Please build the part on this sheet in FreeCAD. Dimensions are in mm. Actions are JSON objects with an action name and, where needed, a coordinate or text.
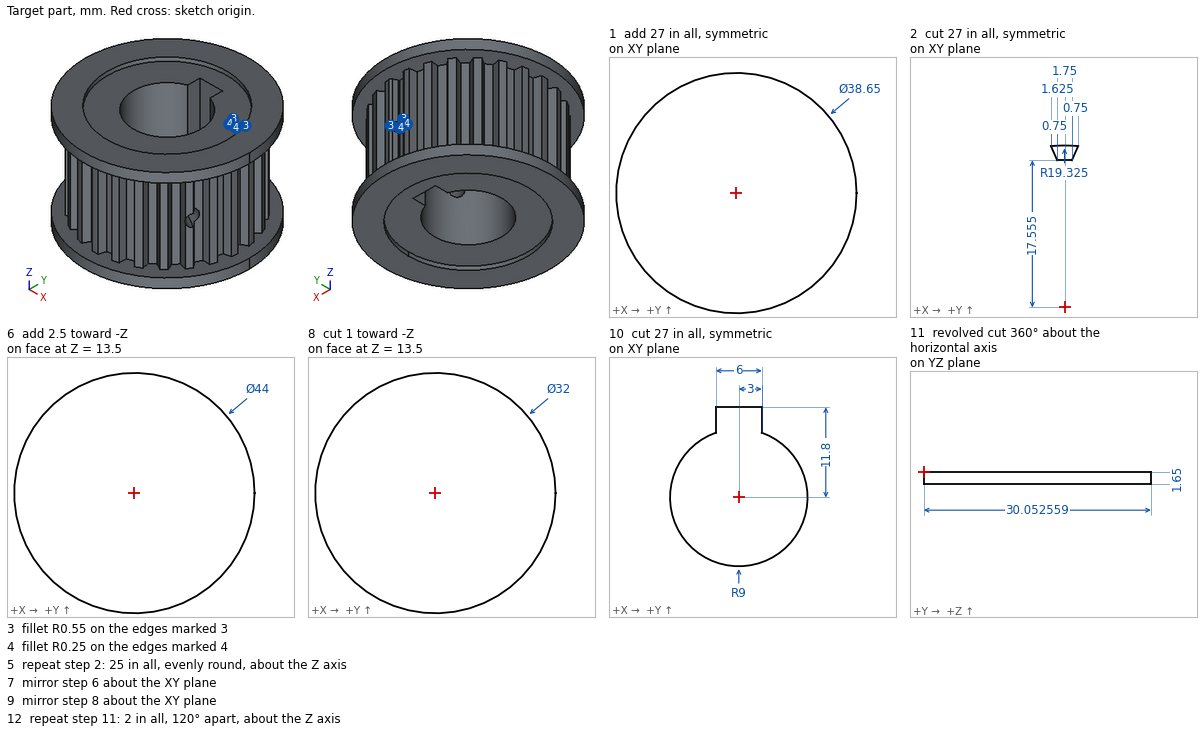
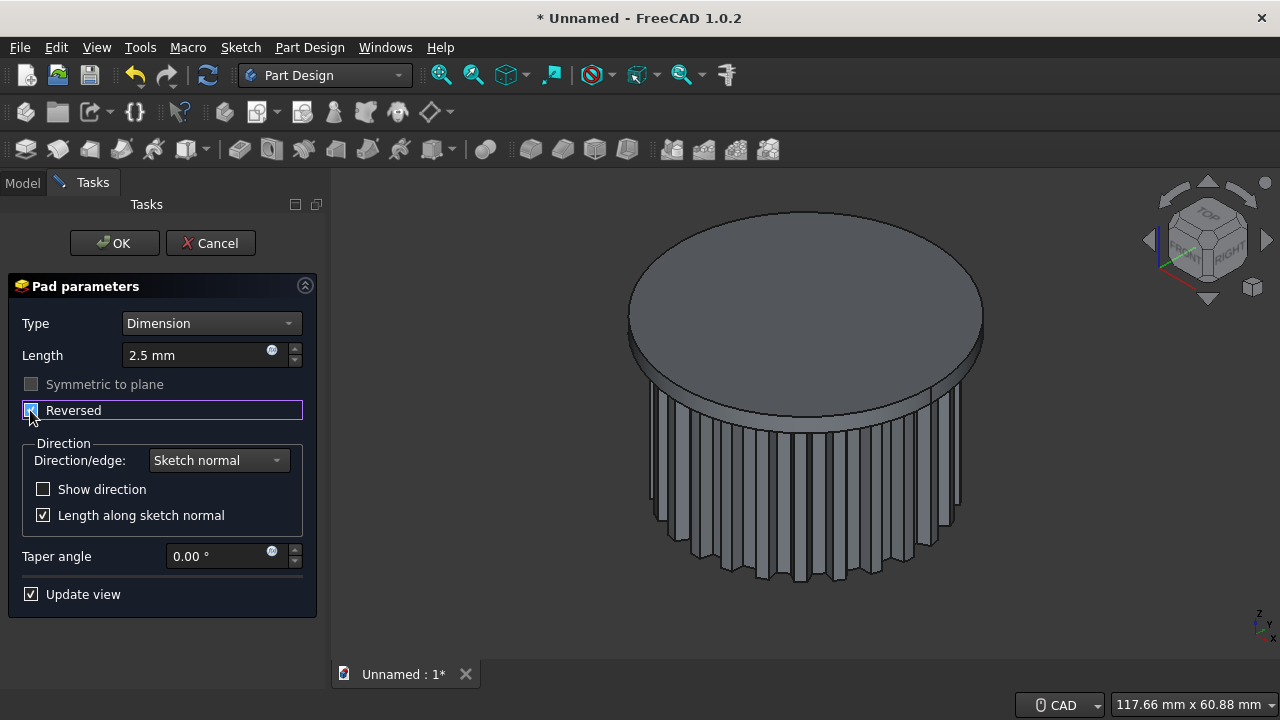
{"action": "left_click", "coordinate": [115, 243]}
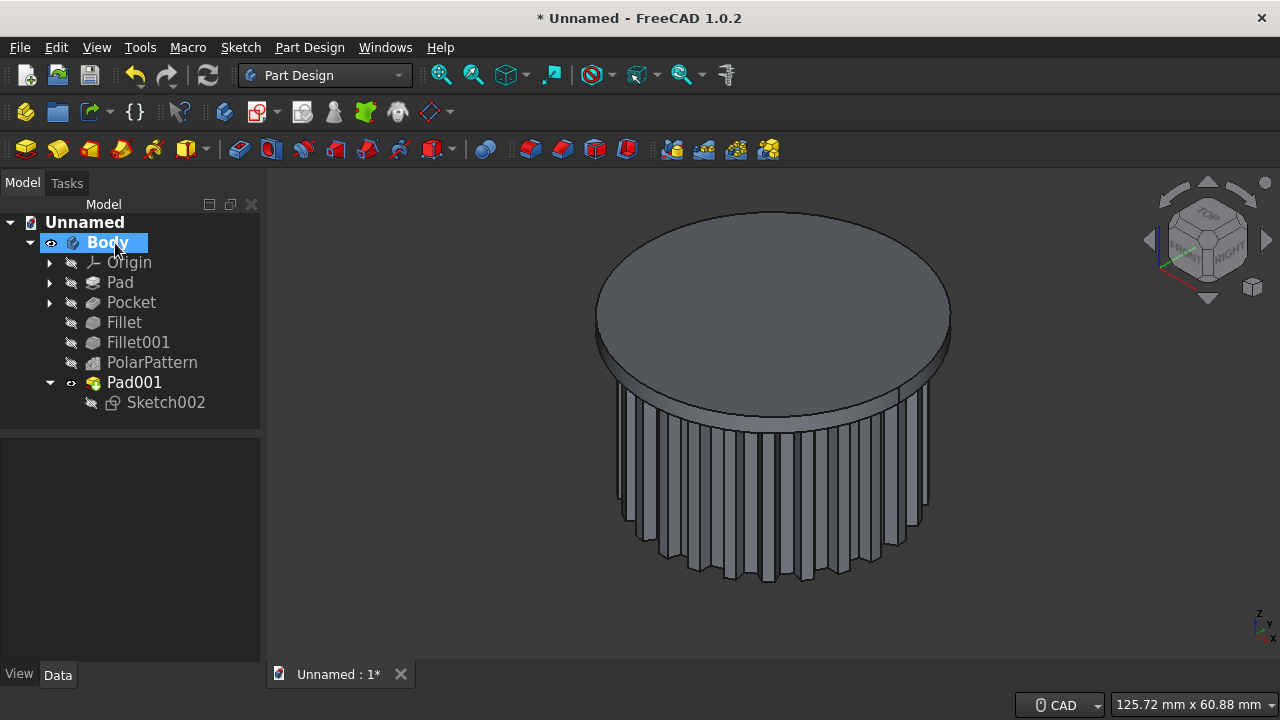
{"action": "left_click", "coordinate": [116, 383]}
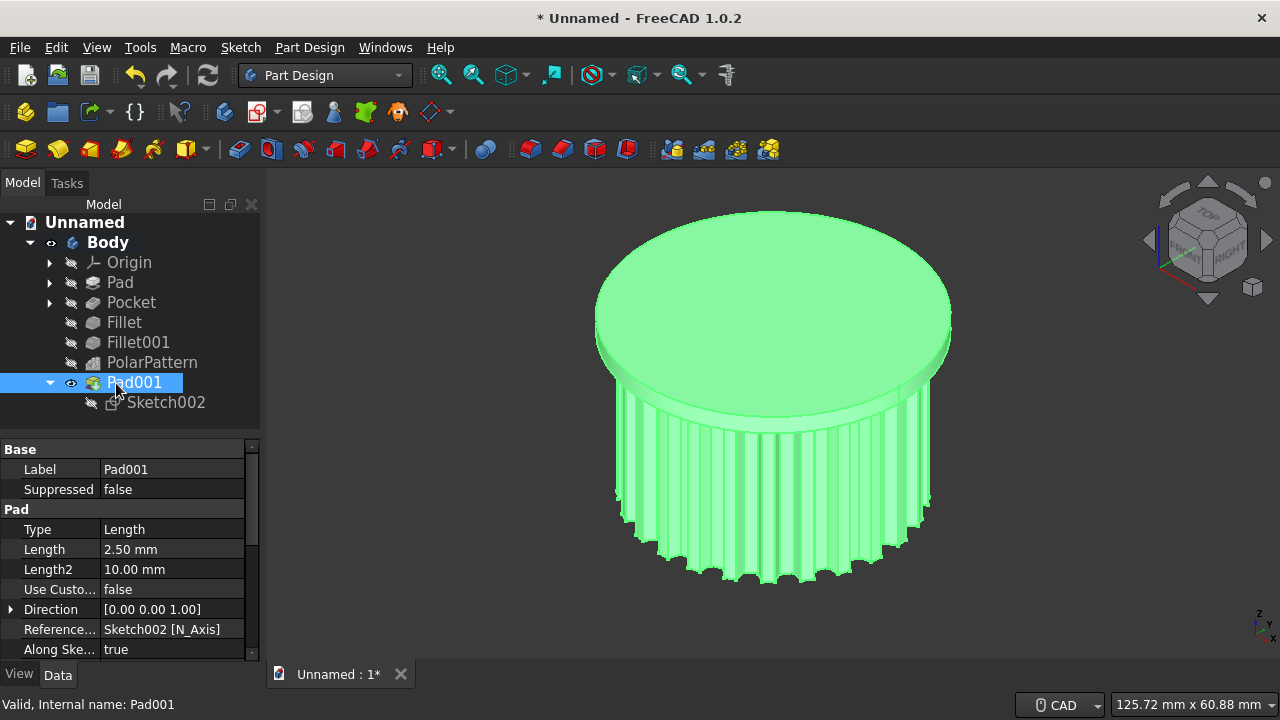
{"action": "left_click", "coordinate": [672, 150]}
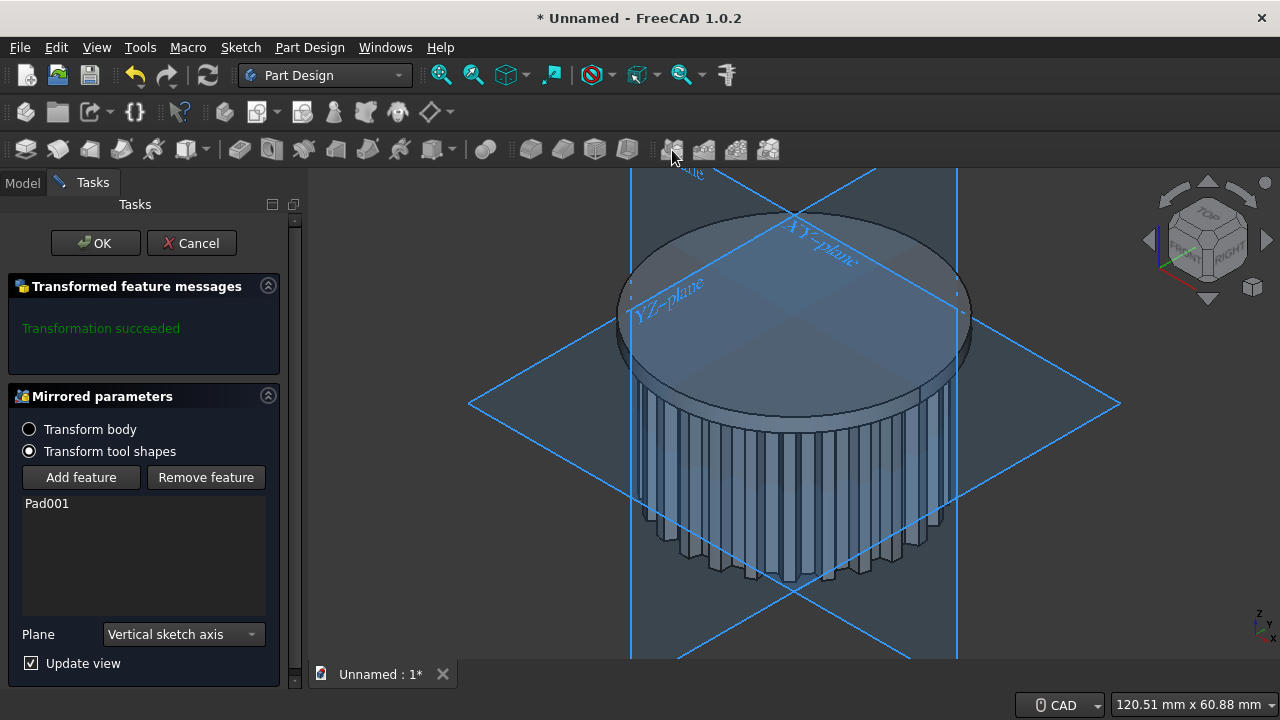
{"action": "left_click", "coordinate": [184, 634]}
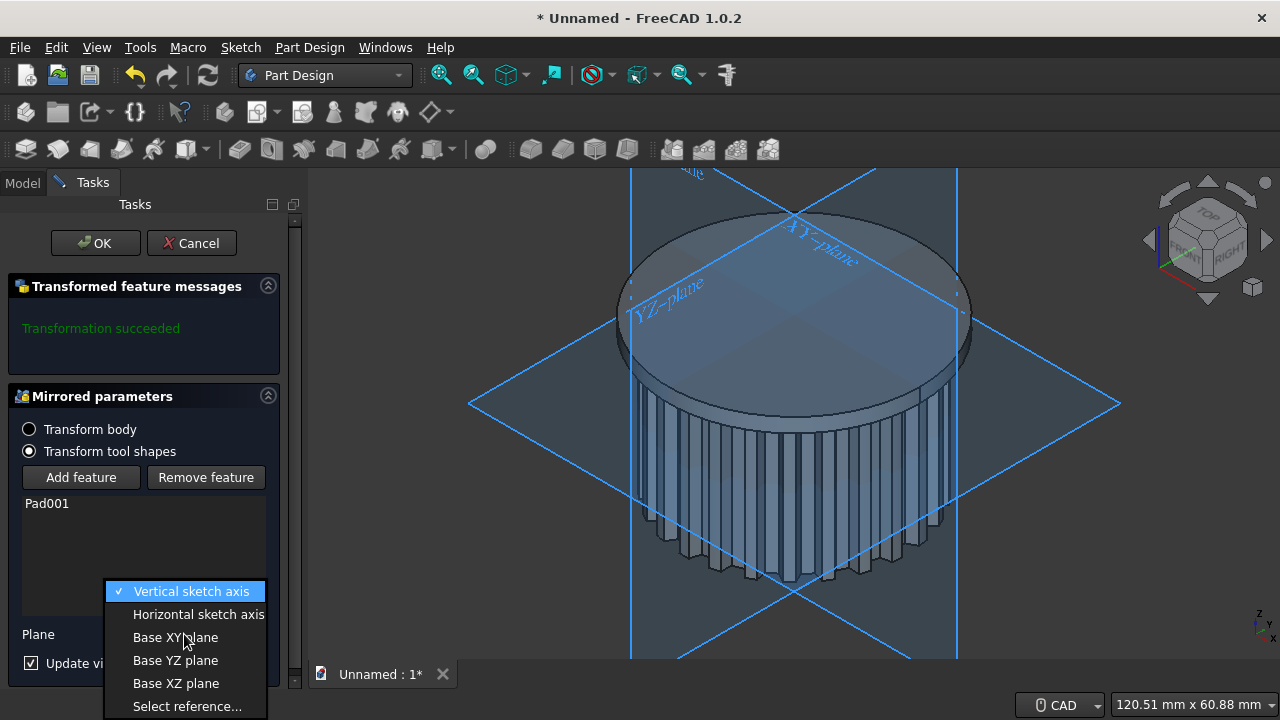
{"action": "left_click", "coordinate": [184, 638]}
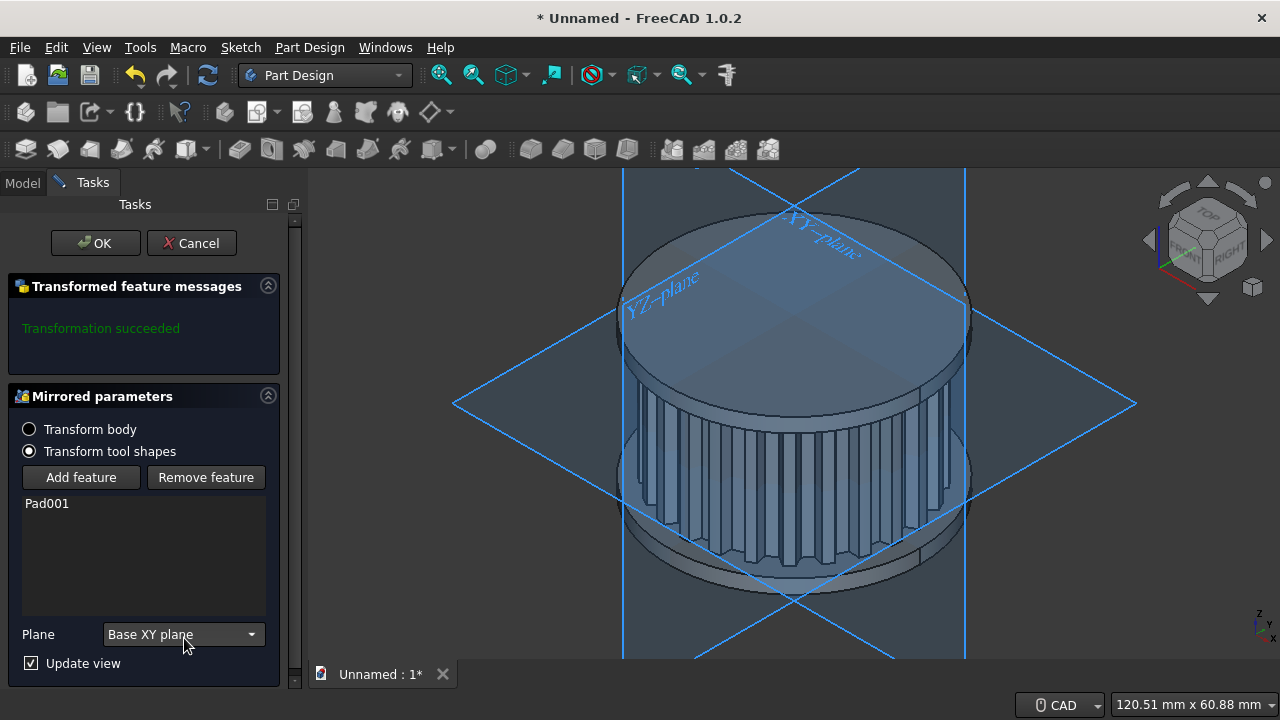
{"action": "left_click", "coordinate": [96, 243]}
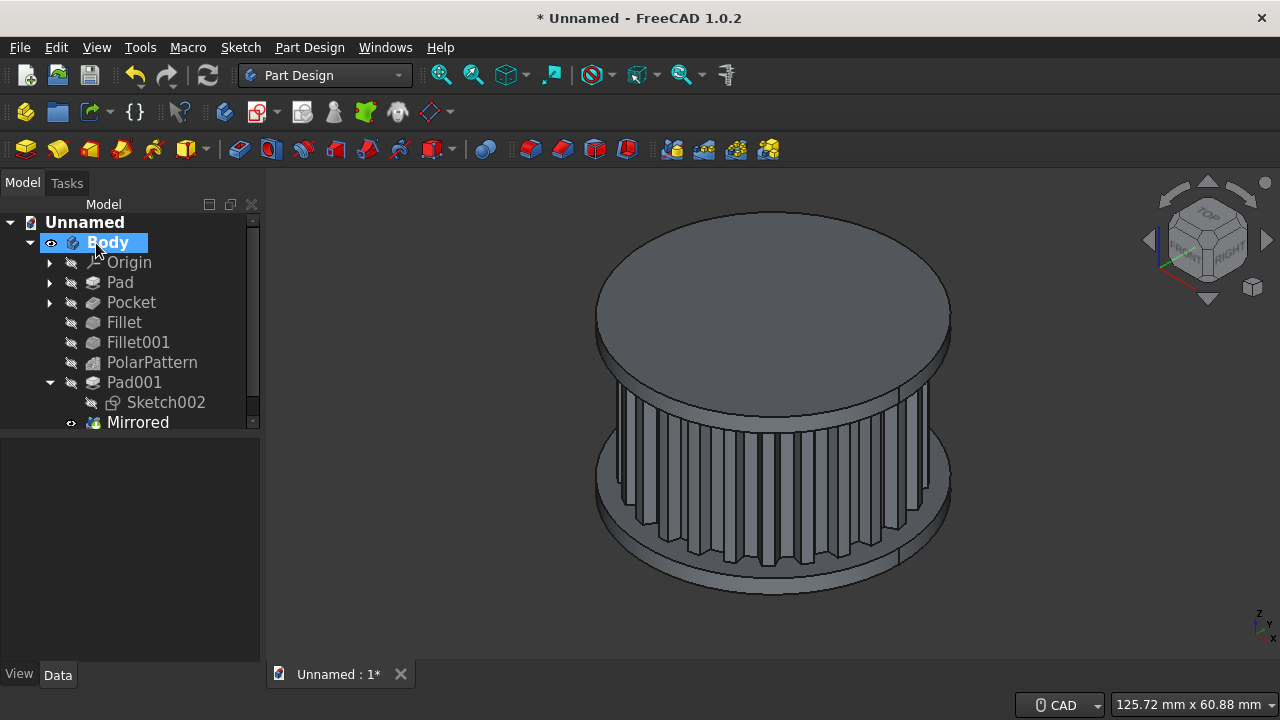
{"action": "left_click", "coordinate": [773, 314]}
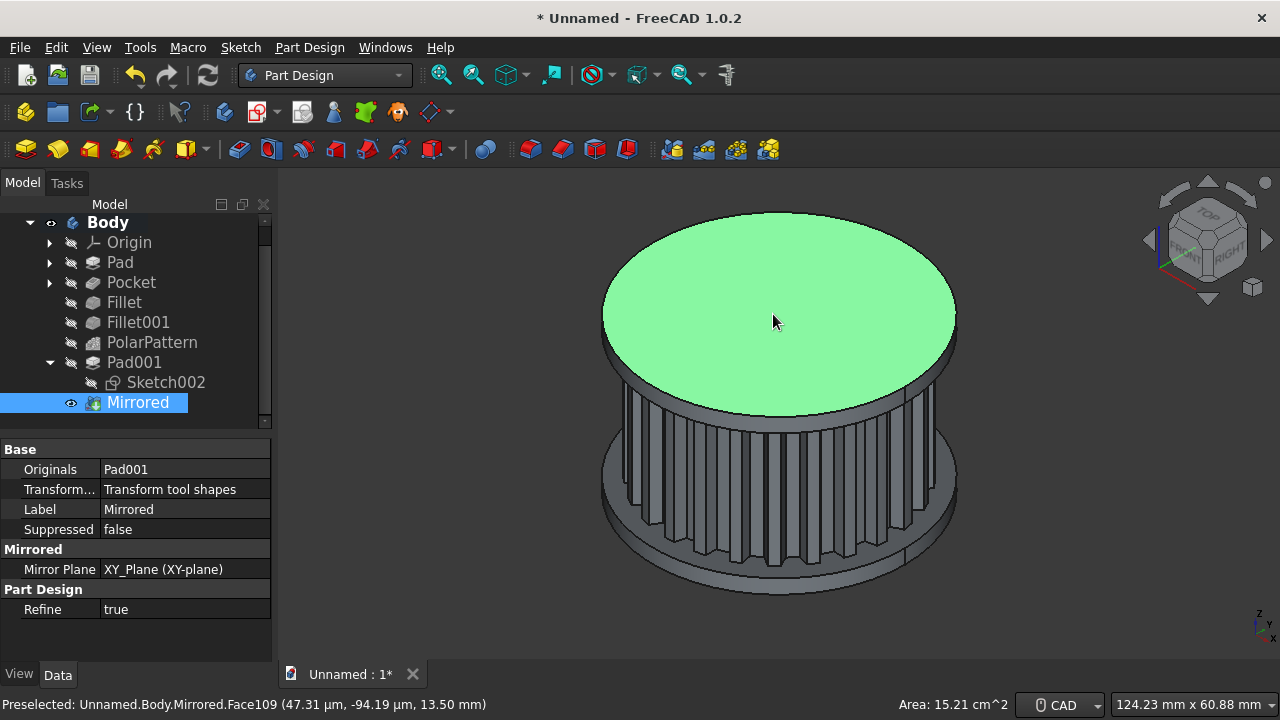
{"action": "left_click", "coordinate": [258, 112]}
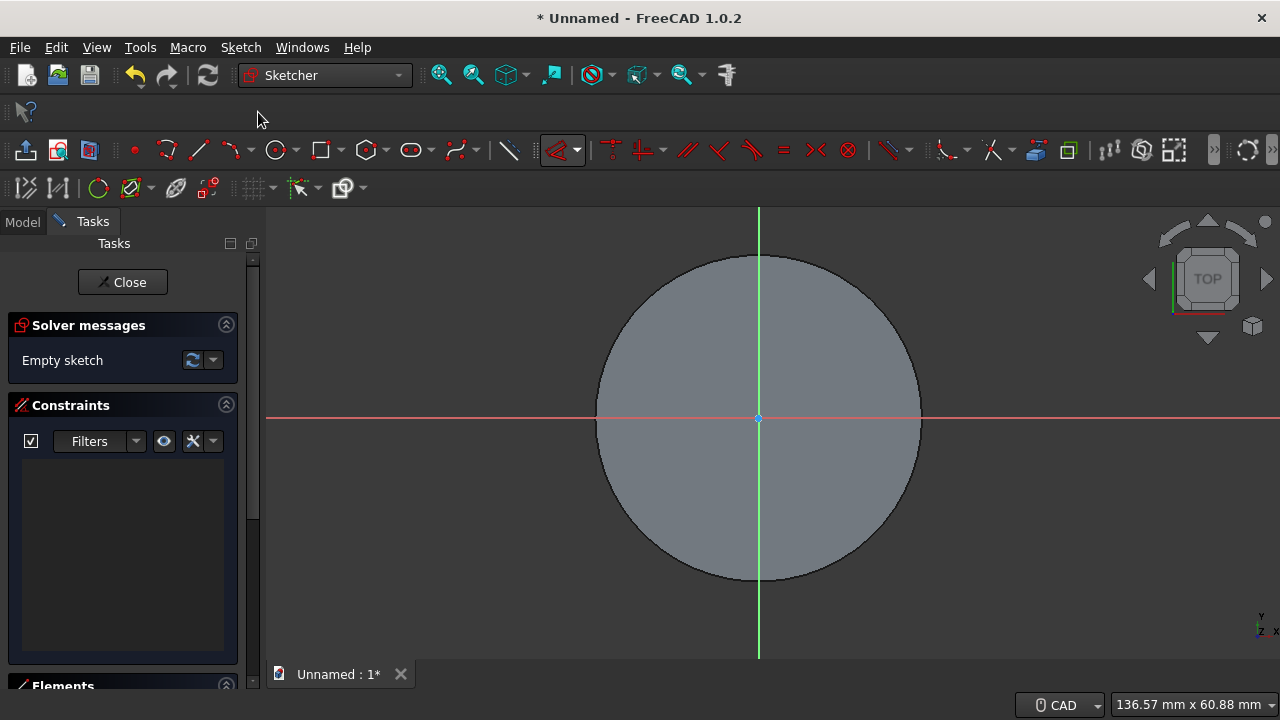
{"action": "left_click", "coordinate": [276, 150]}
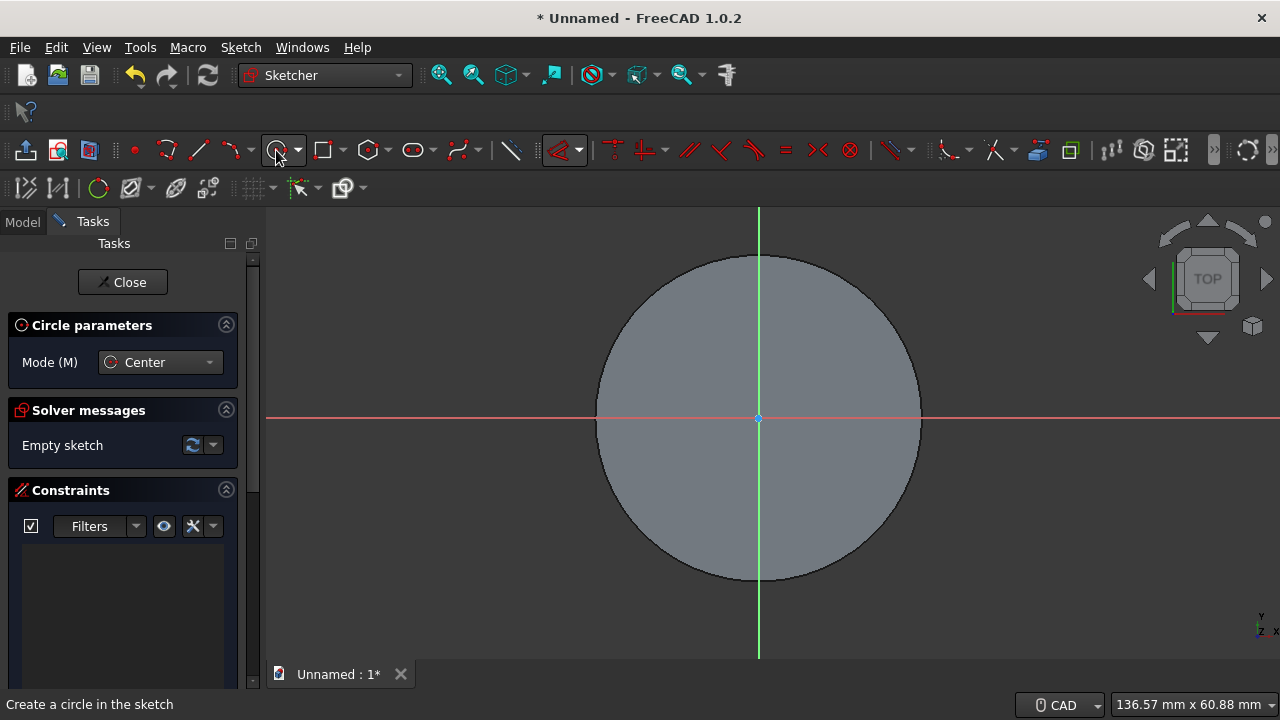
{"action": "left_click", "coordinate": [759, 418]}
{"action": "mouse_move", "coordinate": [843, 334]}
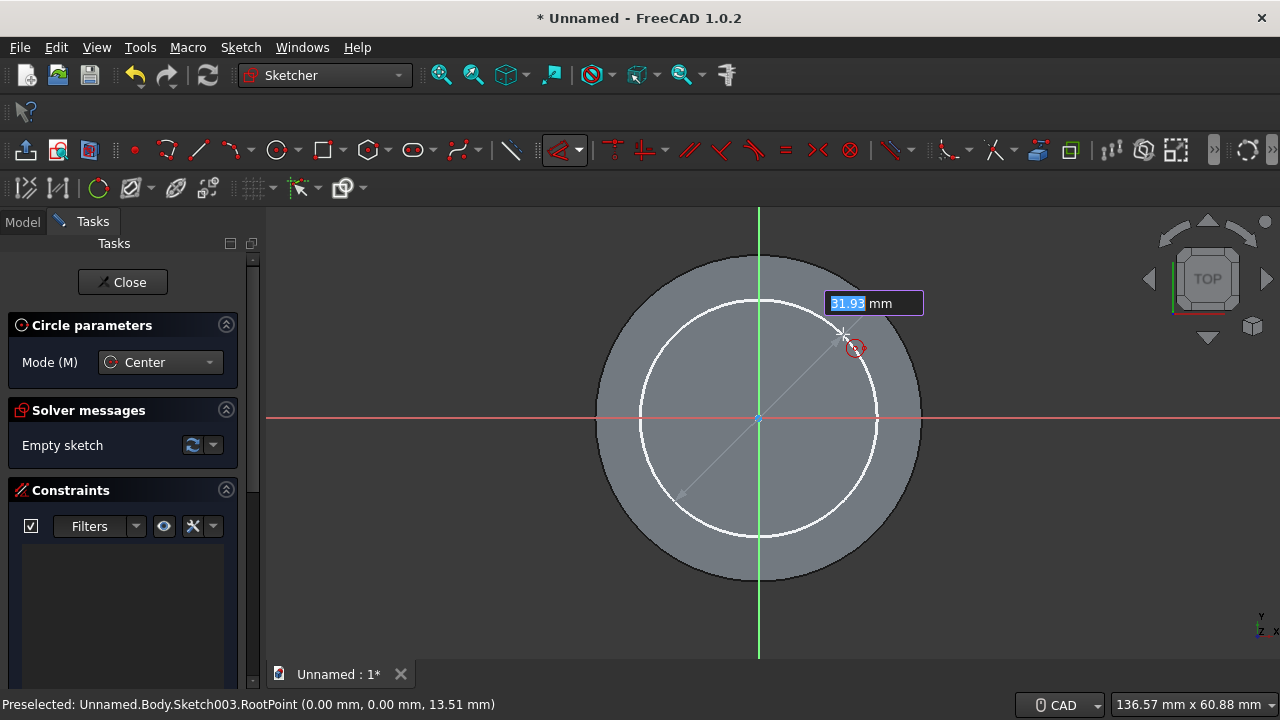
{"action": "type", "text": "32"}
{"action": "key", "text": "Return"}
{"action": "key", "text": "Escape"}